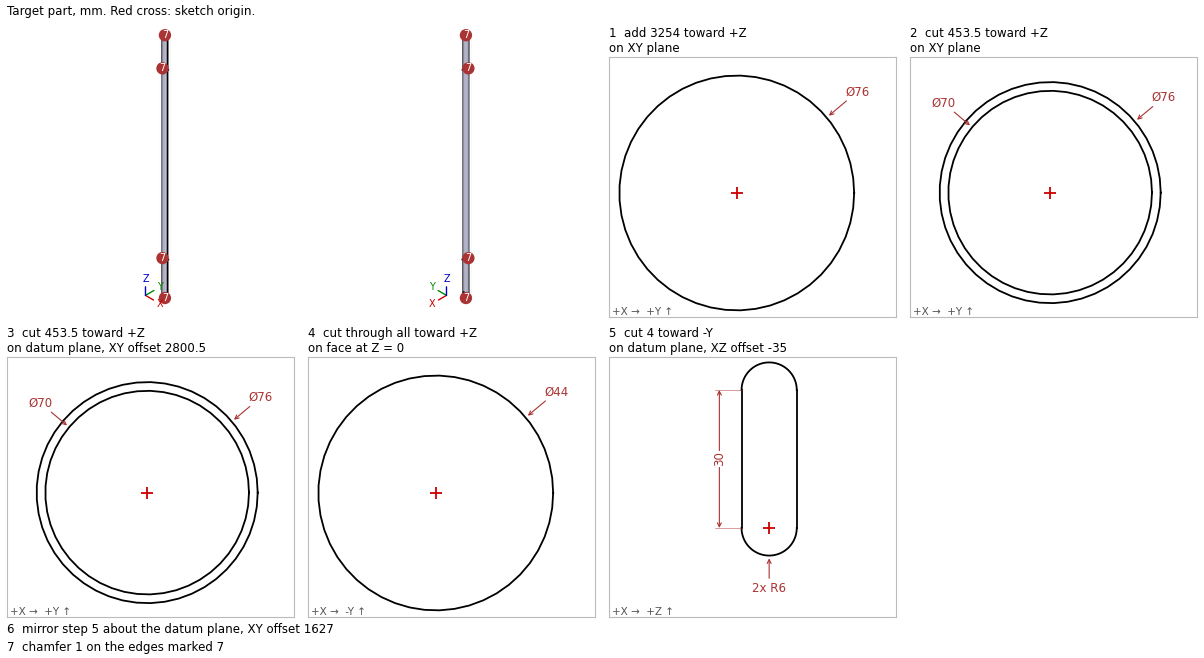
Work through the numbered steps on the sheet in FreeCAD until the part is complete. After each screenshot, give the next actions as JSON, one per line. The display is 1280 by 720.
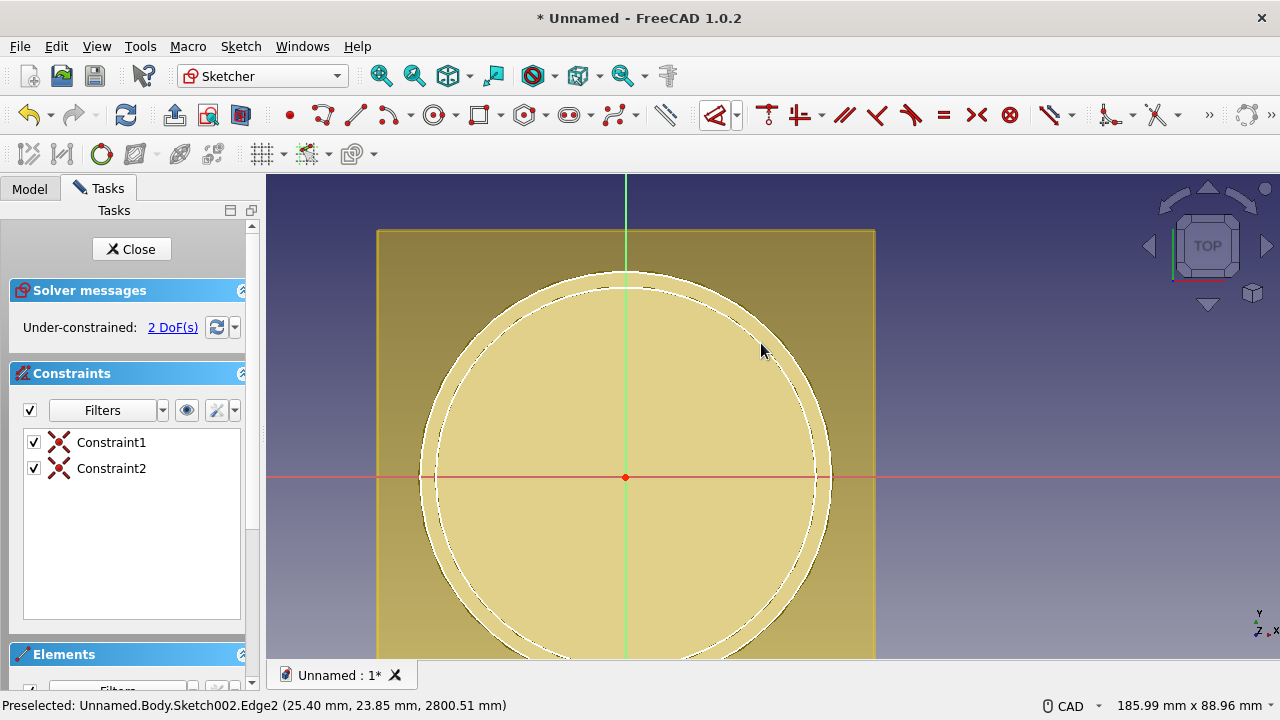
{"action": "left_click", "coordinate": [771, 332]}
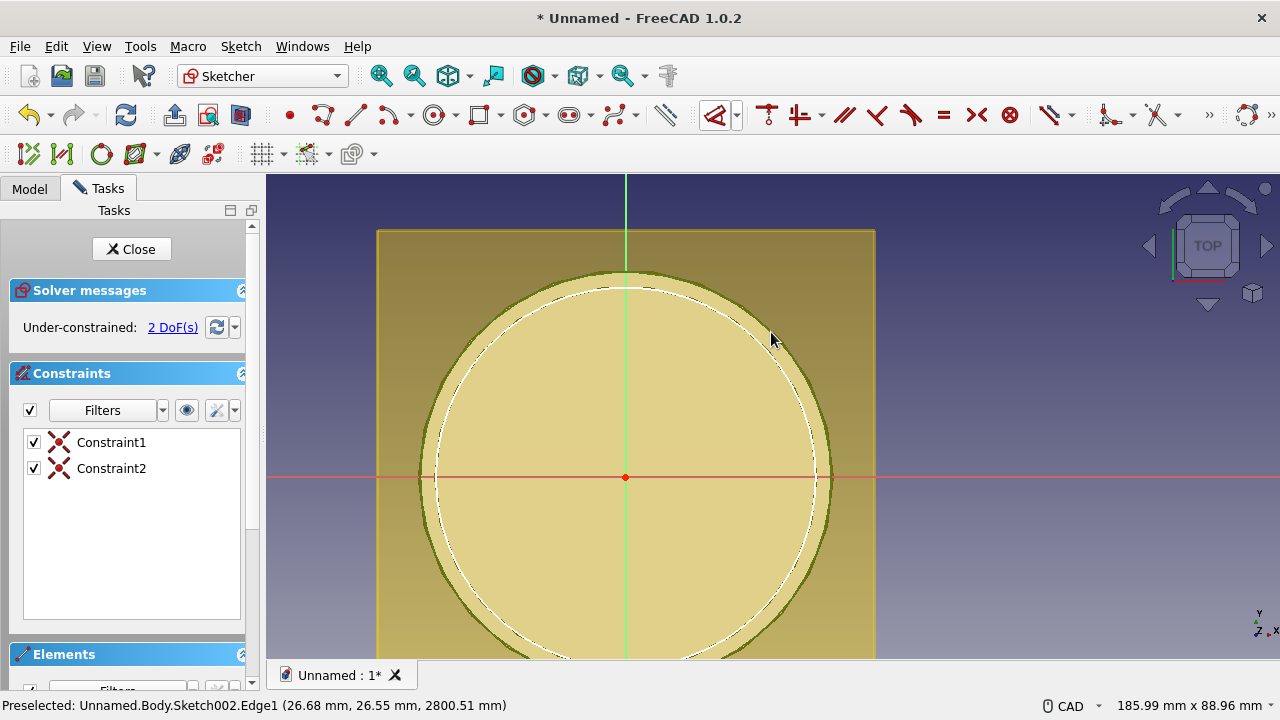
{"action": "key", "text": "k o"}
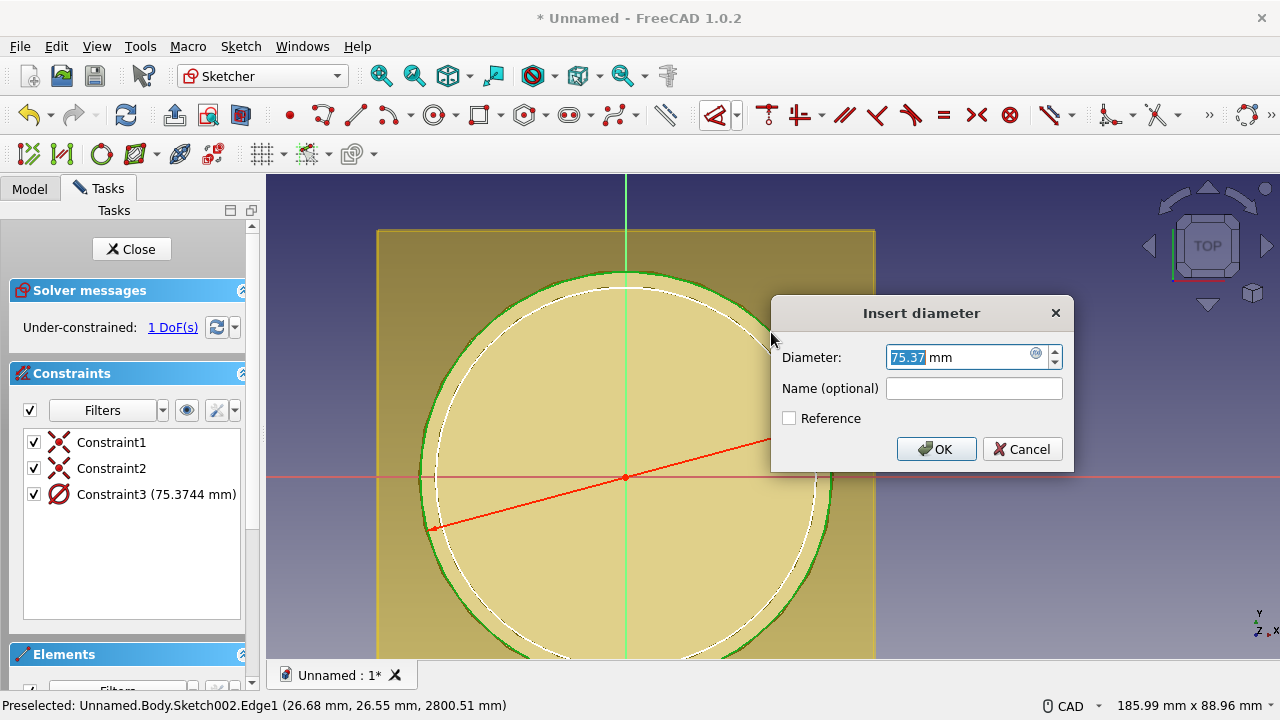
{"action": "type", "text": "76"}
{"action": "key", "text": "Return"}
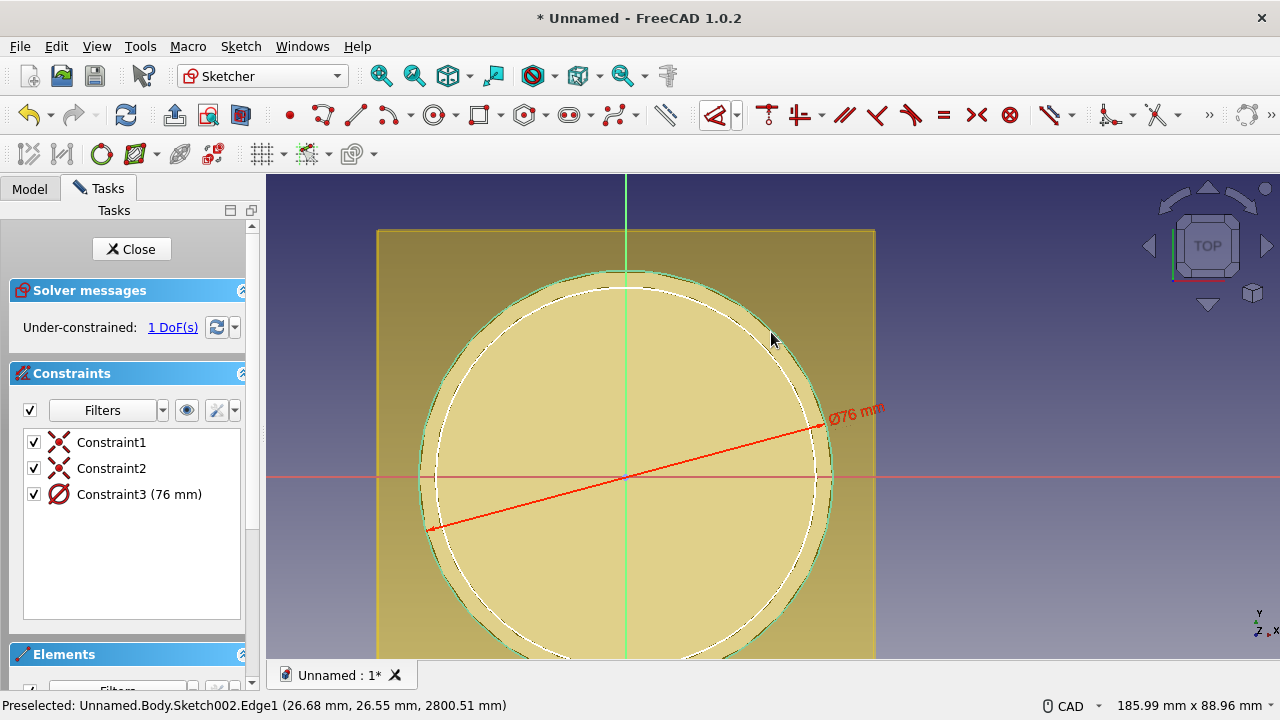
{"action": "left_click", "coordinate": [760, 343]}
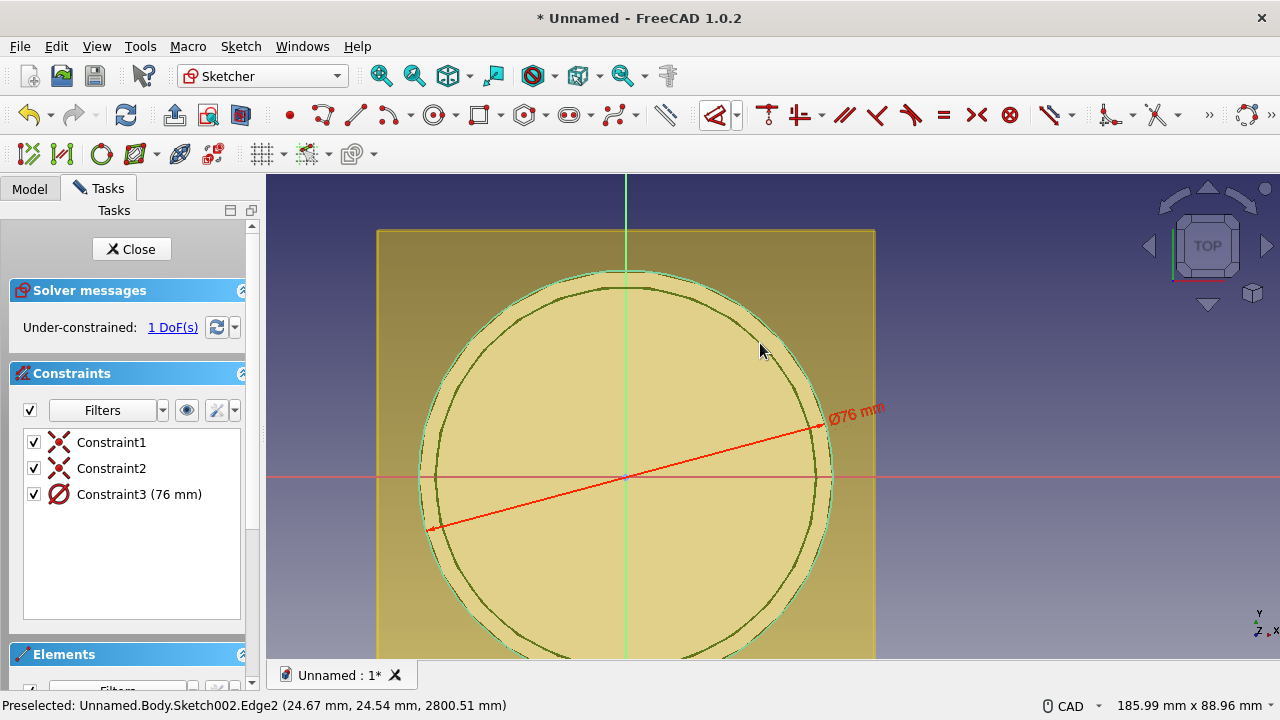
{"action": "key", "text": "k o"}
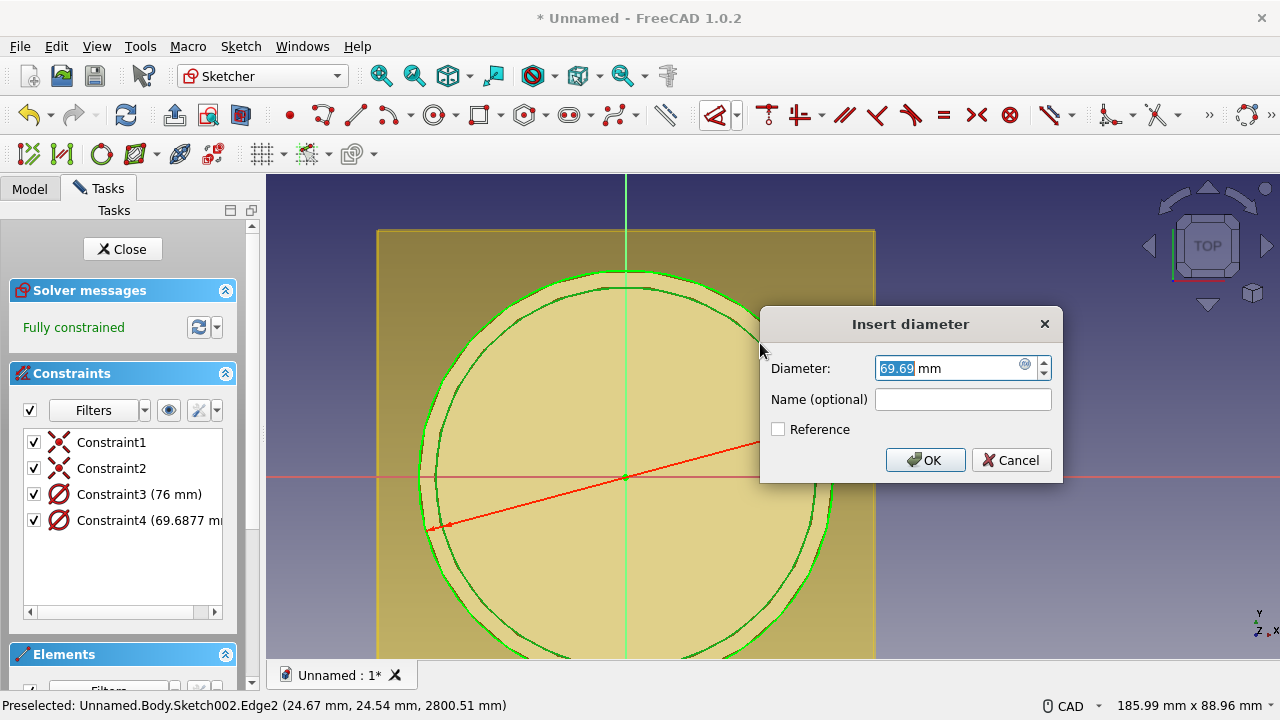
{"action": "type", "text": "70"}
{"action": "key", "text": "Return"}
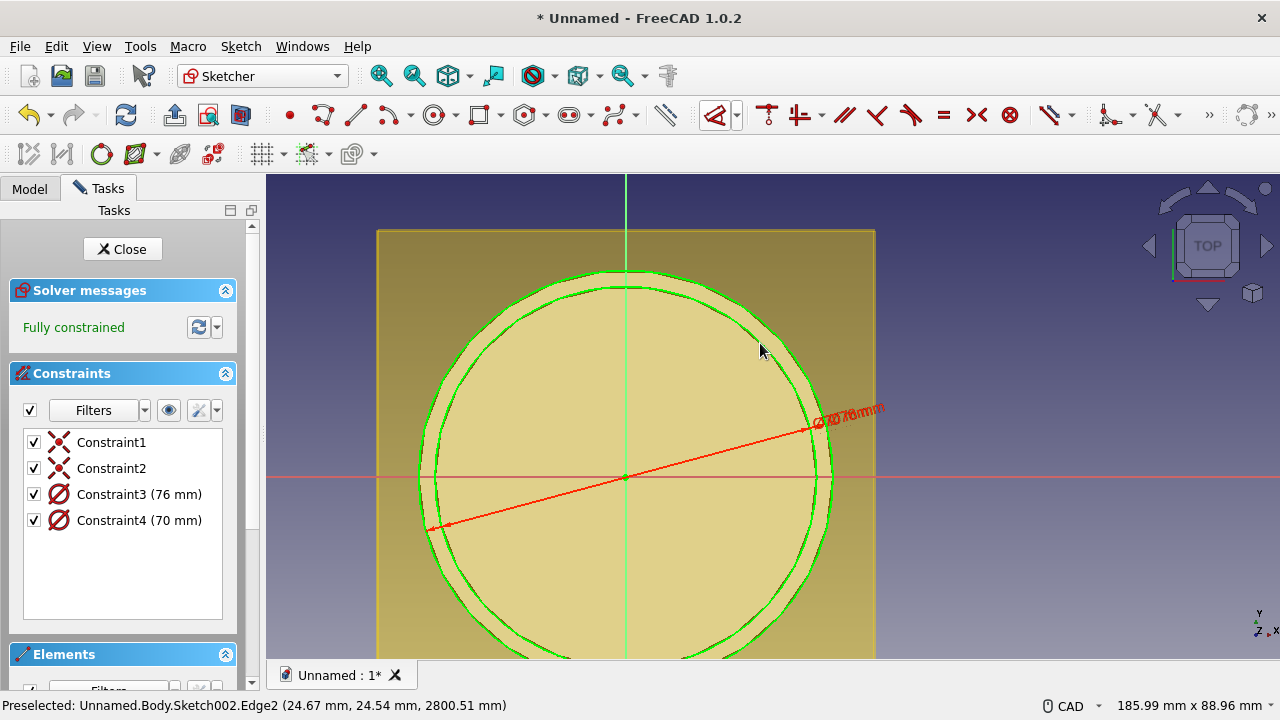
{"action": "left_click", "coordinate": [123, 249]}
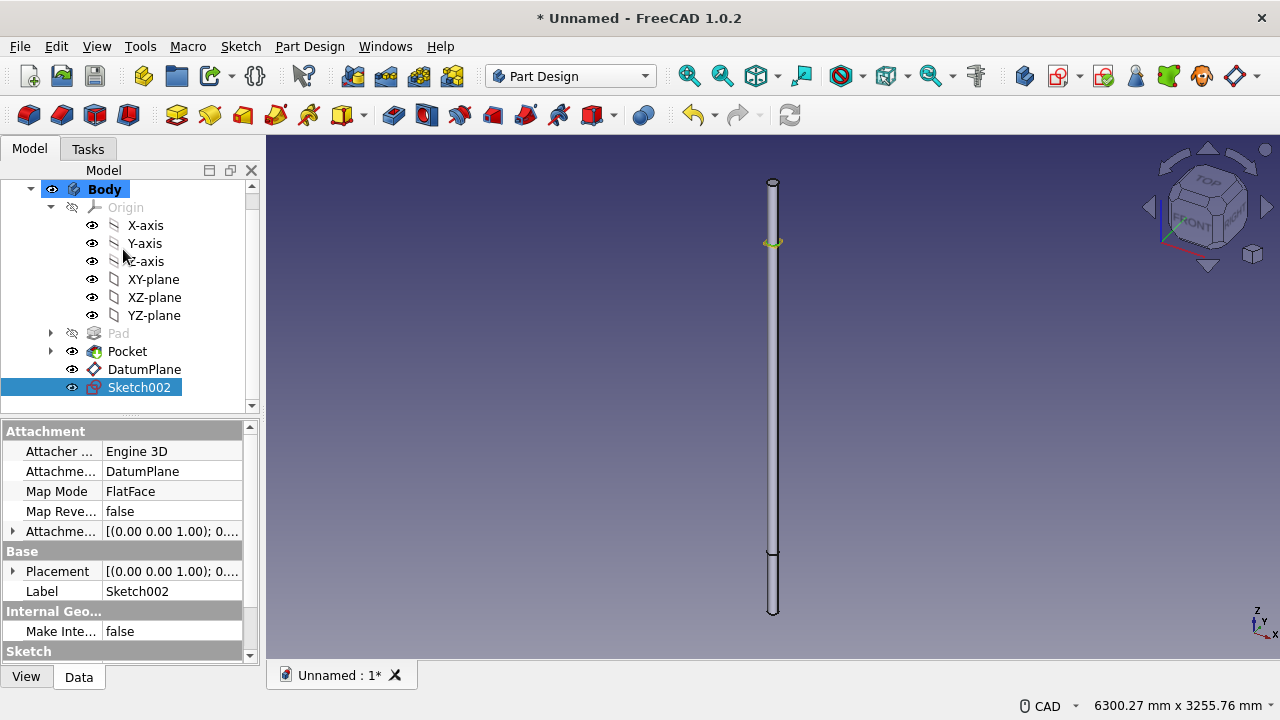
{"action": "left_click", "coordinate": [394, 116]}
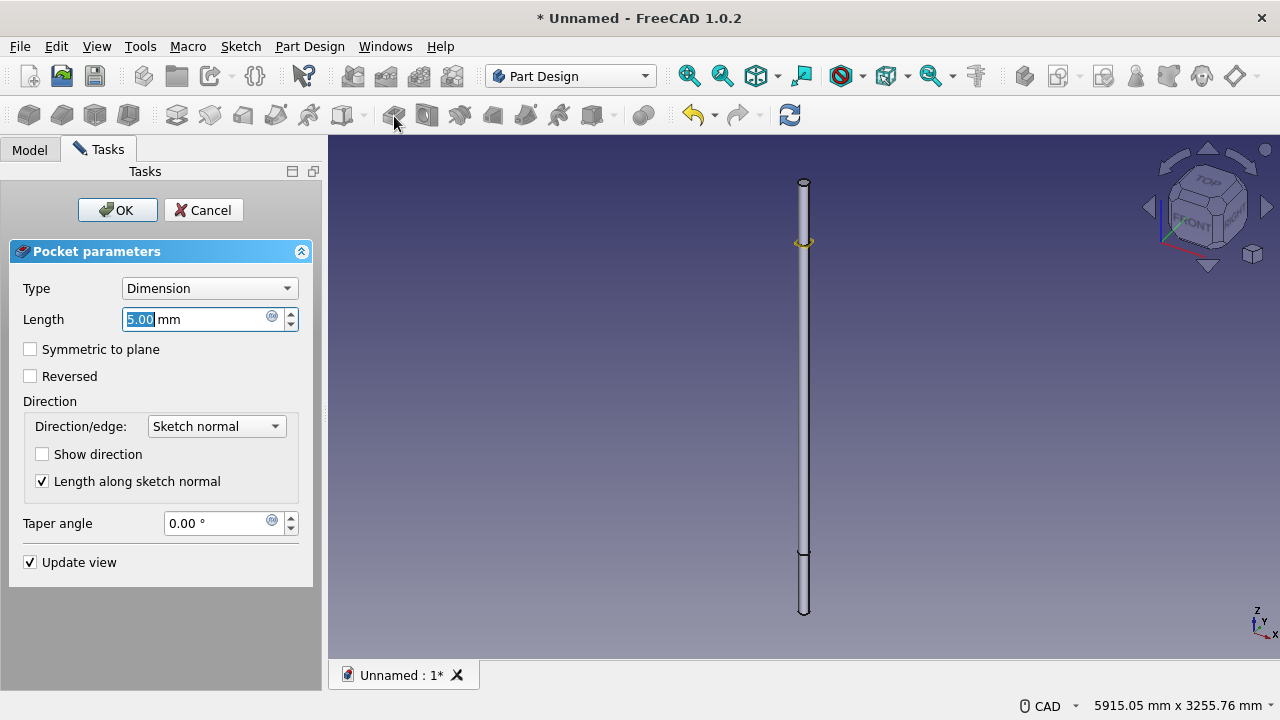
{"action": "type", "text": "453.5"}
{"action": "key", "text": "Tab"}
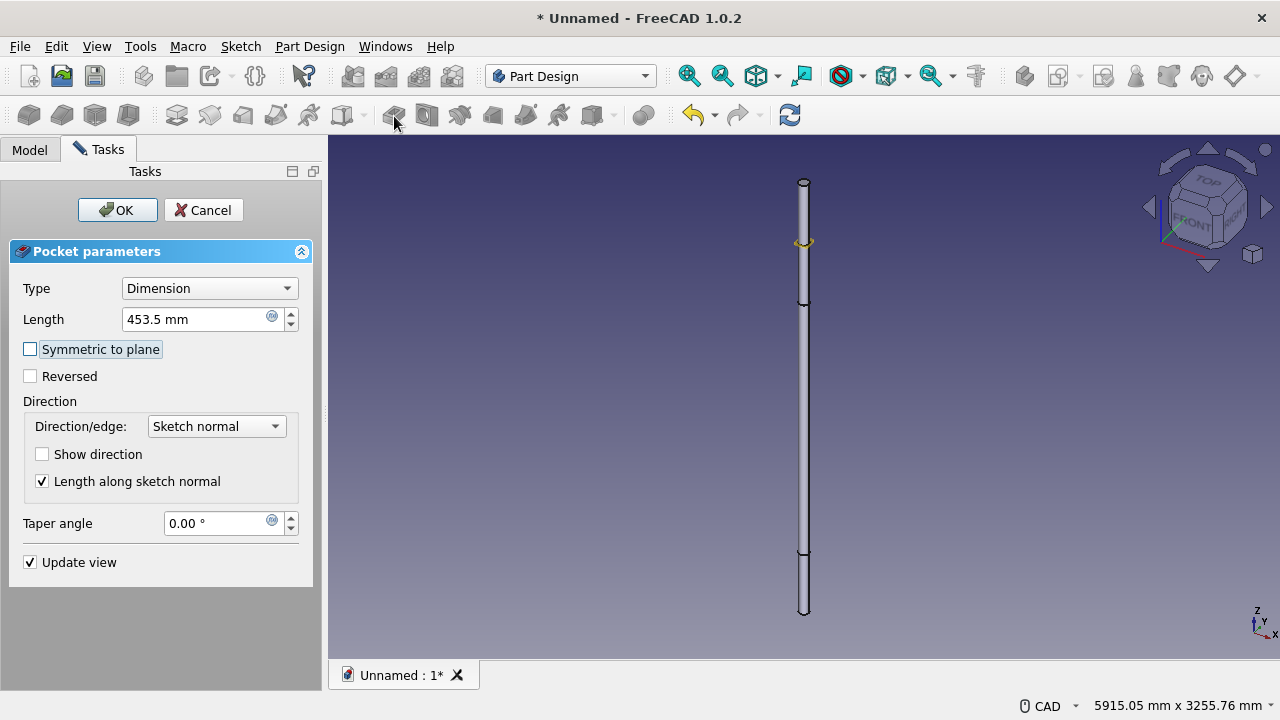
{"action": "left_click", "coordinate": [31, 376]}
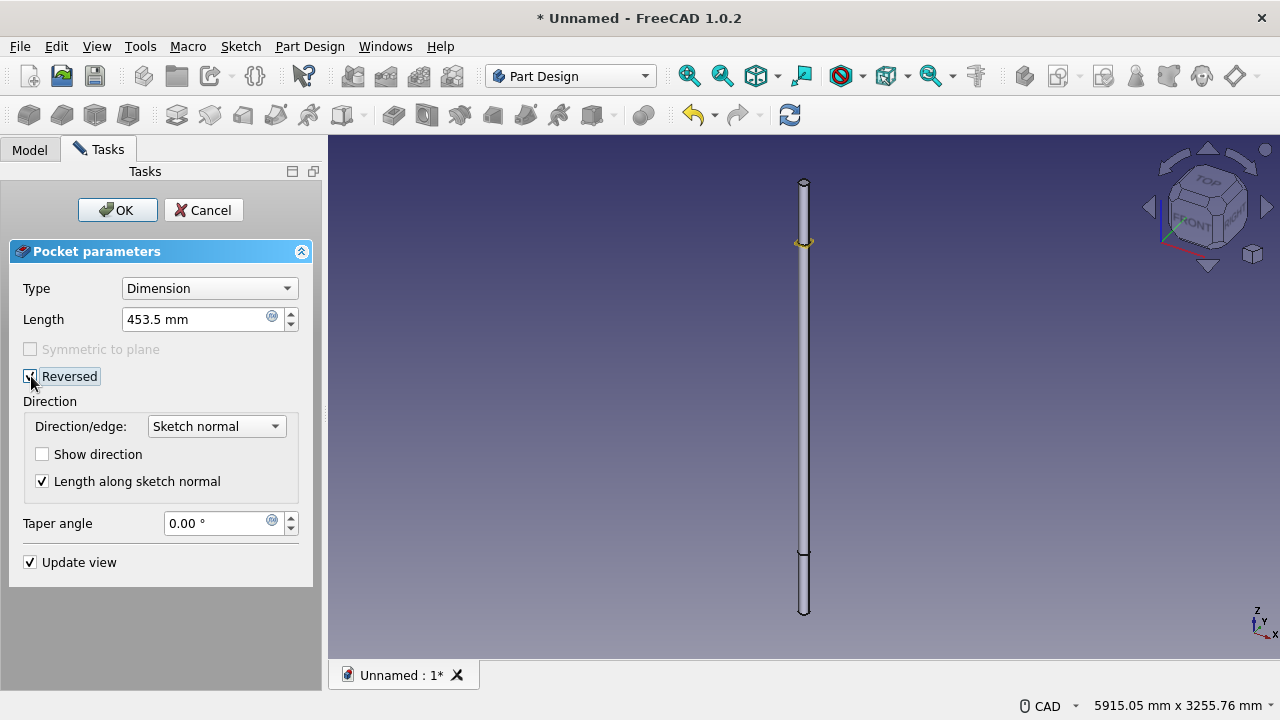
{"action": "left_click", "coordinate": [118, 210]}